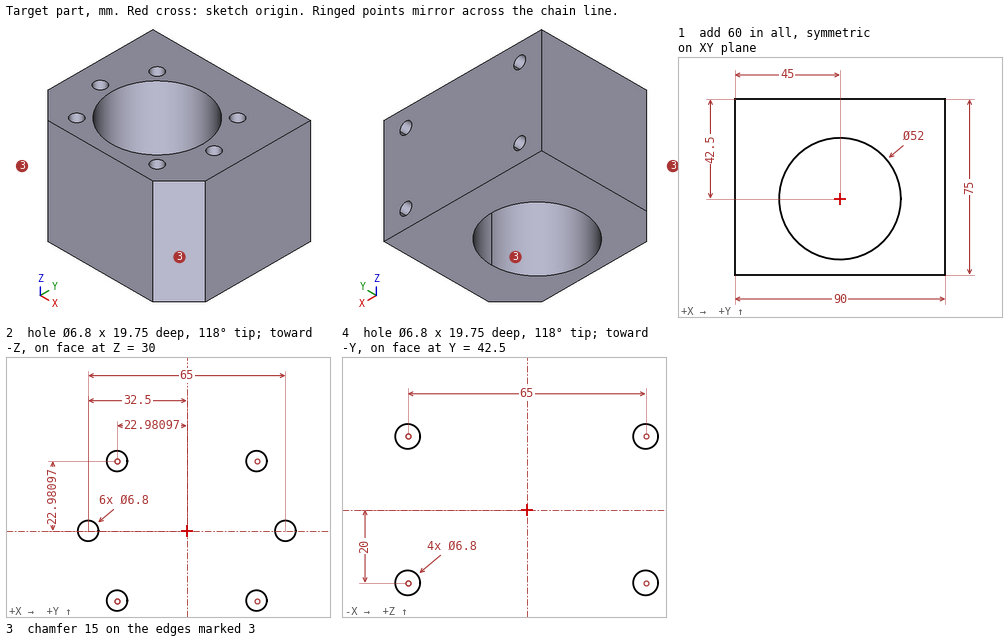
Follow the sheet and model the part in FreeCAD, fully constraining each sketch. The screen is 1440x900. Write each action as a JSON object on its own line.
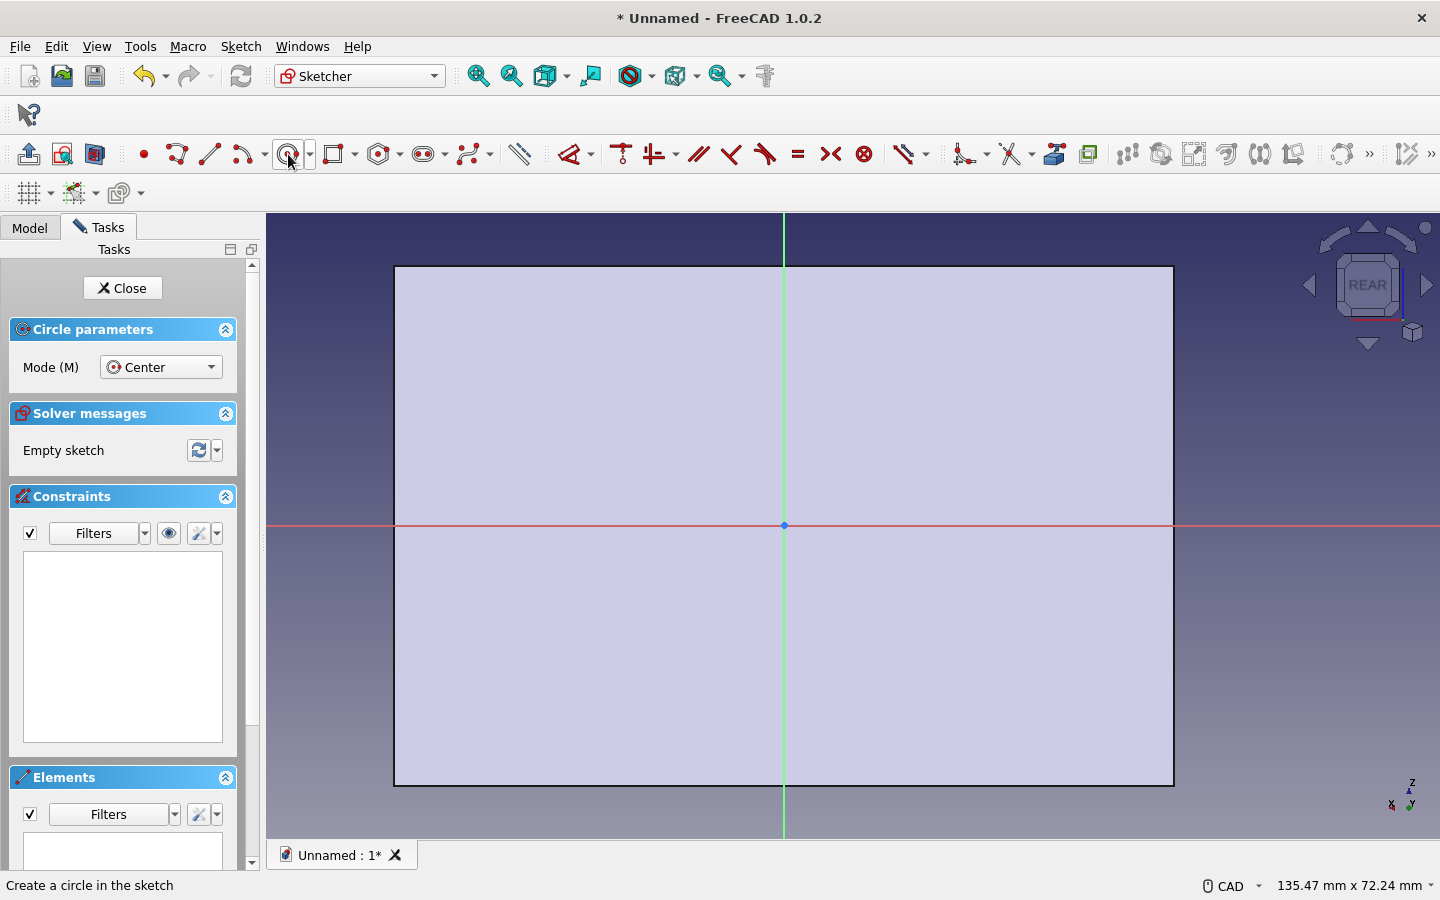
{"action": "left_click", "coordinate": [503, 699]}
{"action": "mouse_move", "coordinate": [523, 678]}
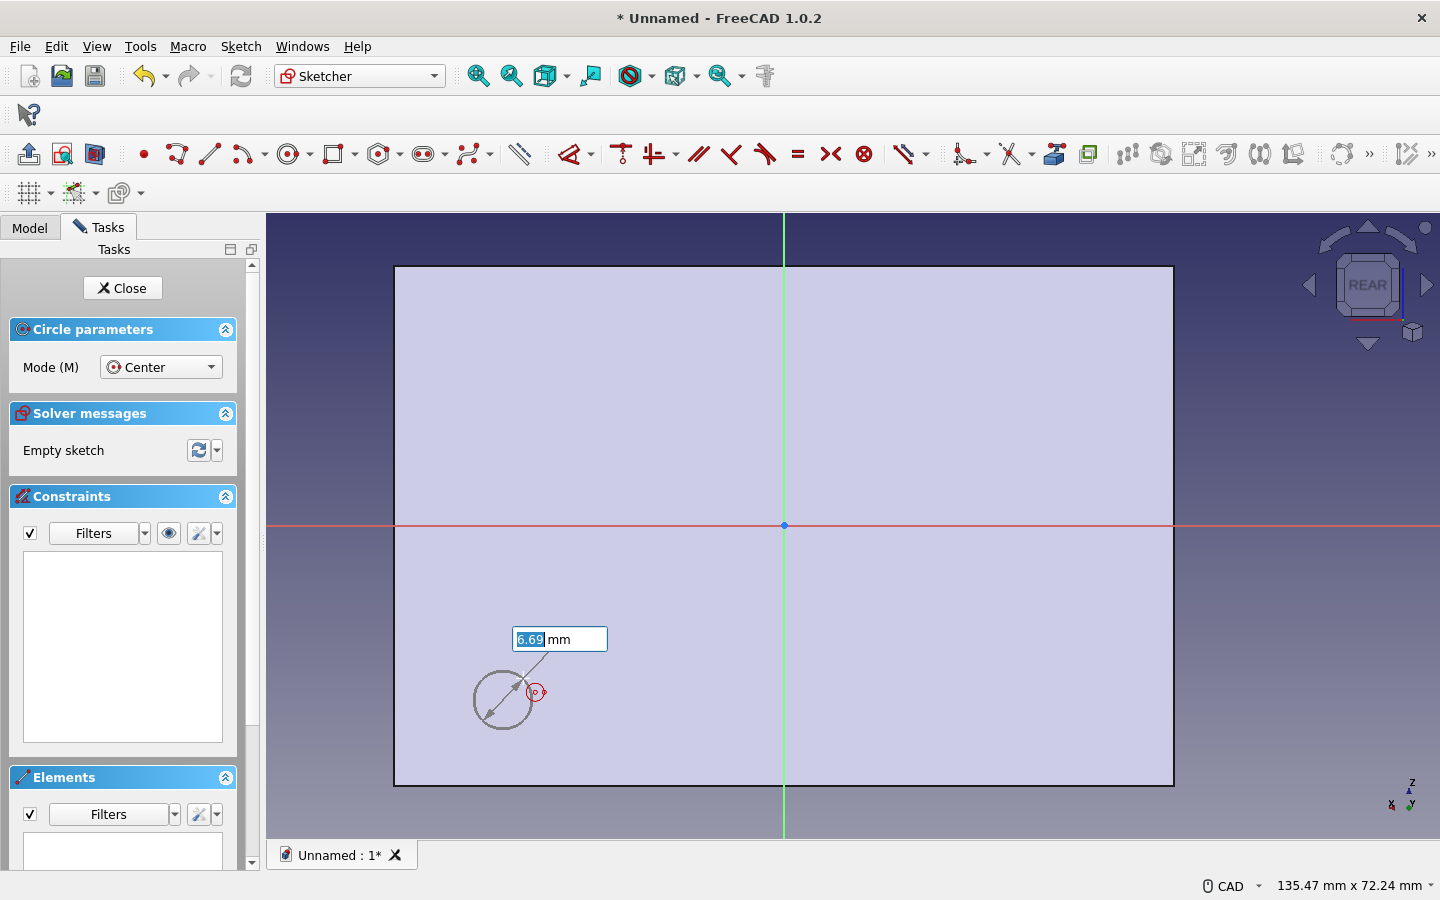
{"action": "type", "text": "6.8"}
{"action": "key", "text": "Return"}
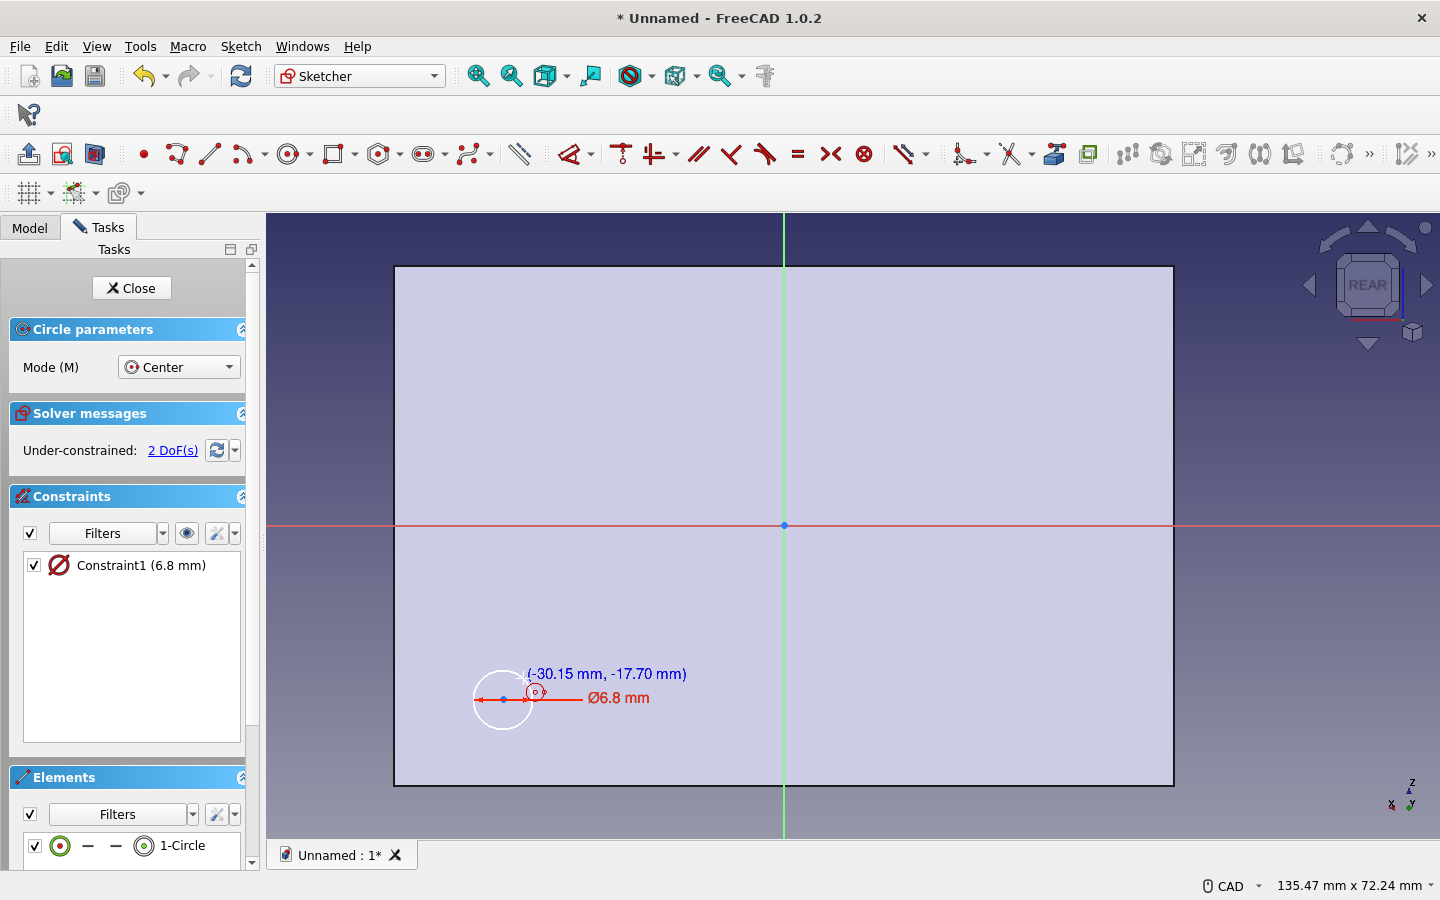
{"action": "left_click", "coordinate": [503, 352]}
{"action": "mouse_move", "coordinate": [523, 331]}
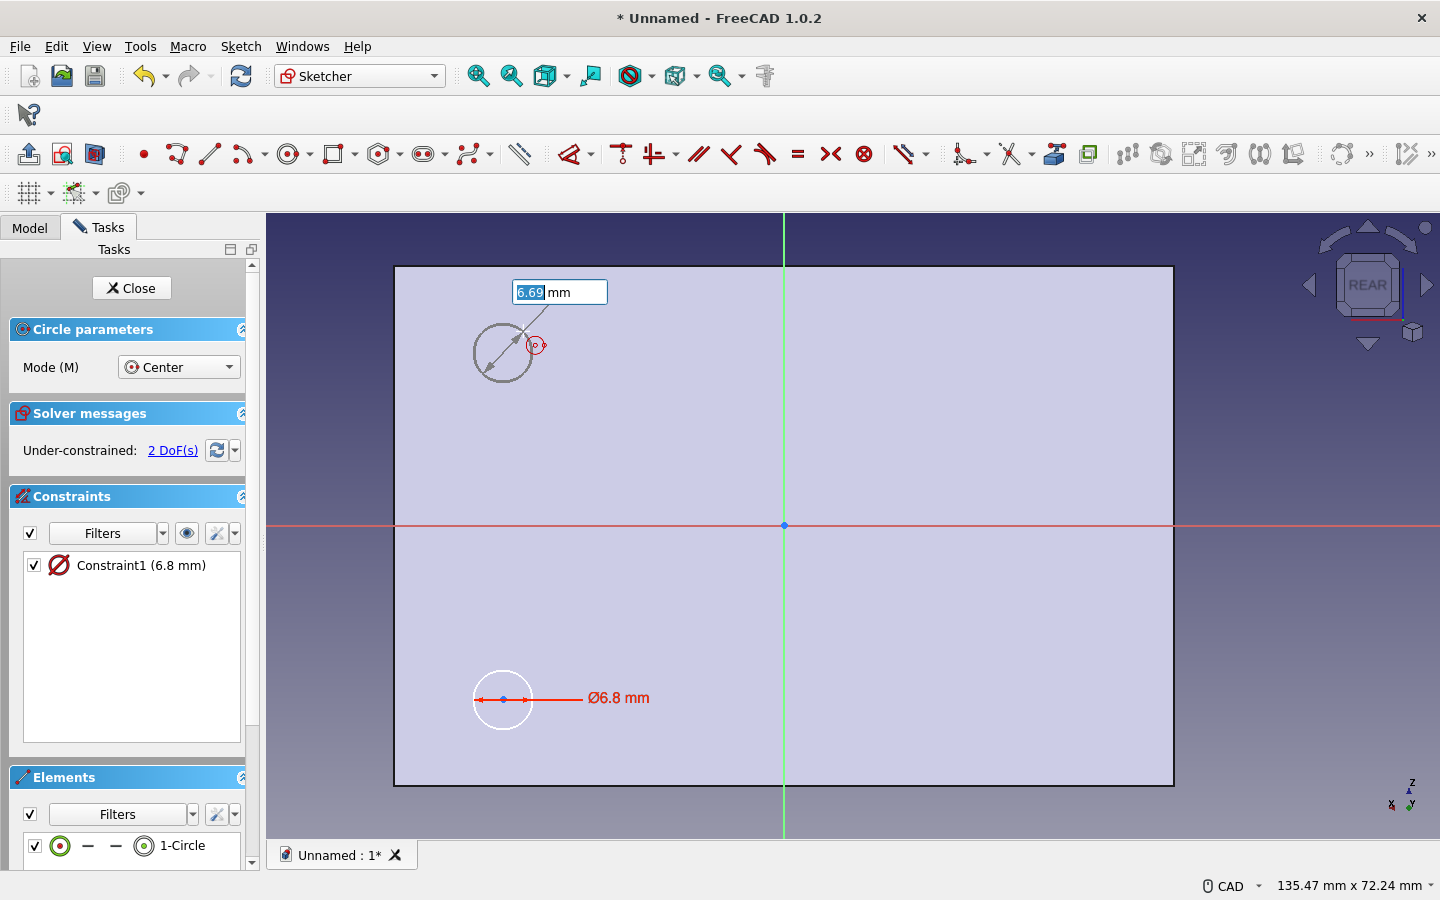
{"action": "type", "text": "6.8"}
{"action": "key", "text": "Return"}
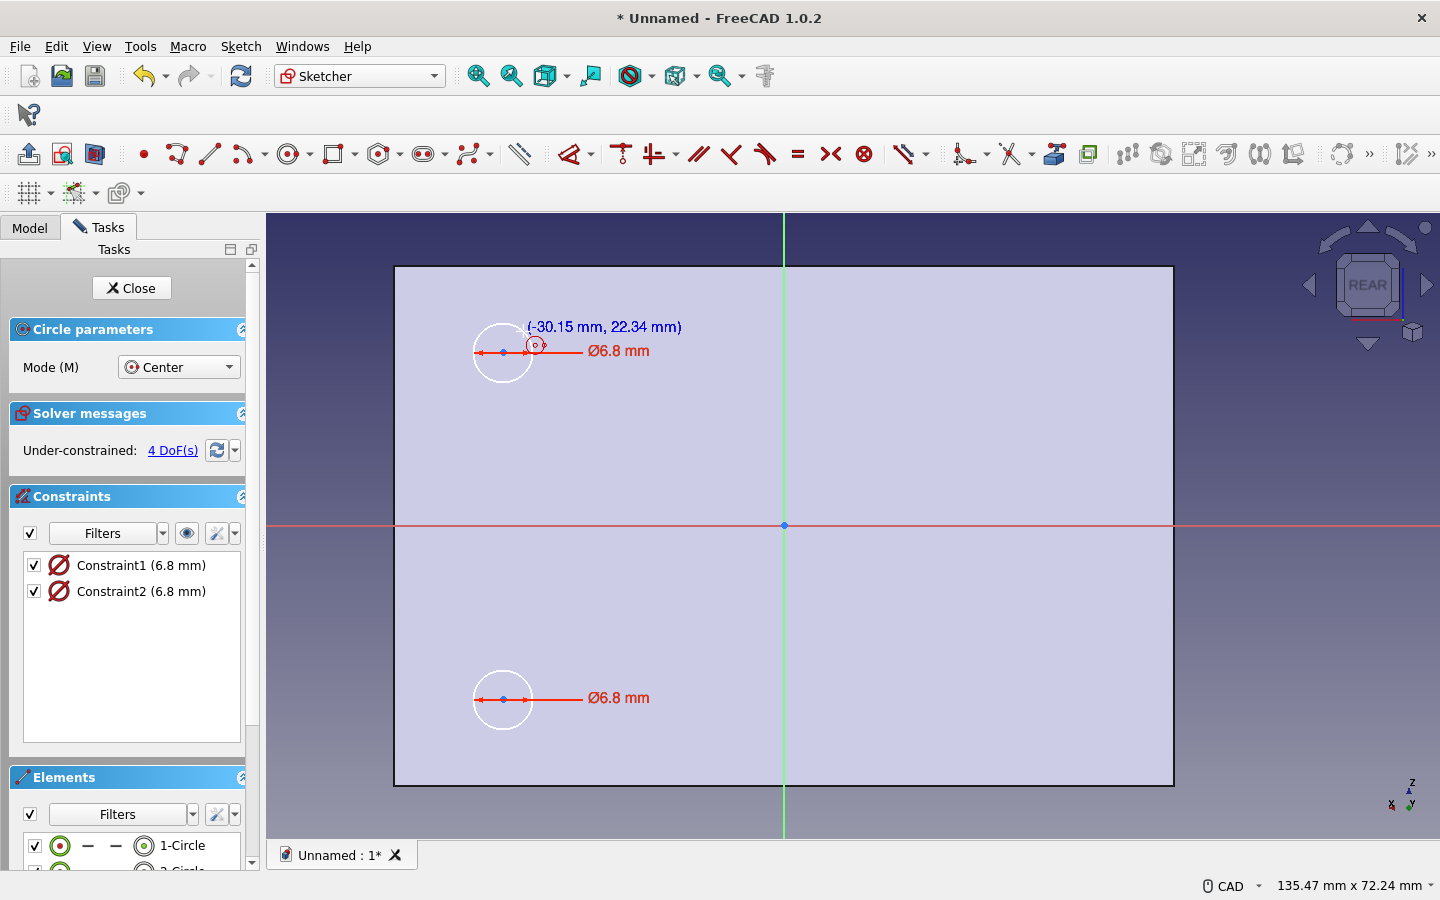
{"action": "left_click", "coordinate": [1066, 352]}
{"action": "mouse_move", "coordinate": [1087, 331]}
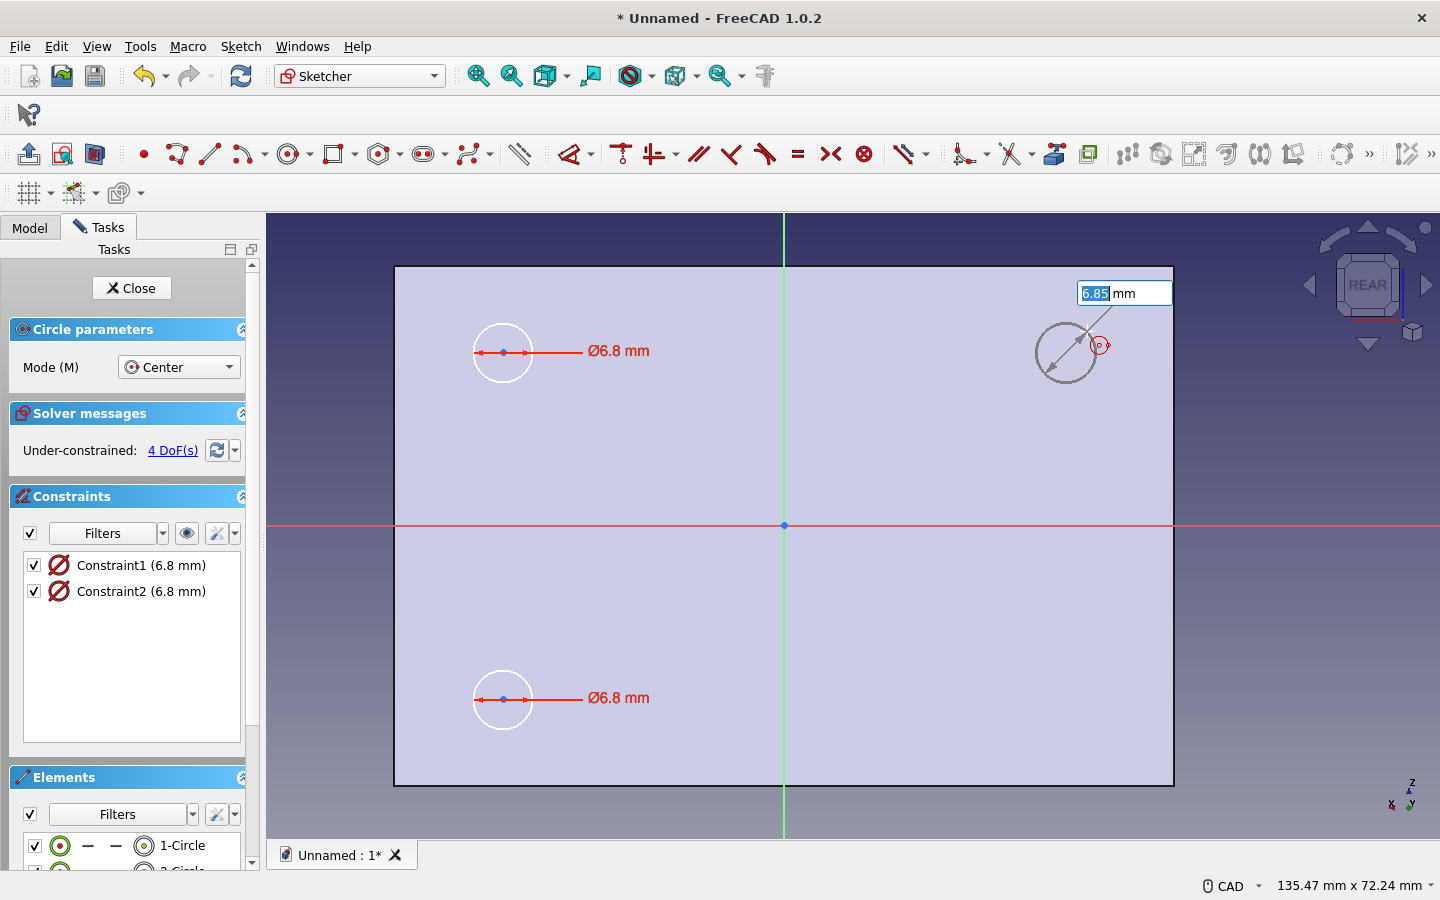
{"action": "type", "text": "6.8"}
{"action": "key", "text": "Return"}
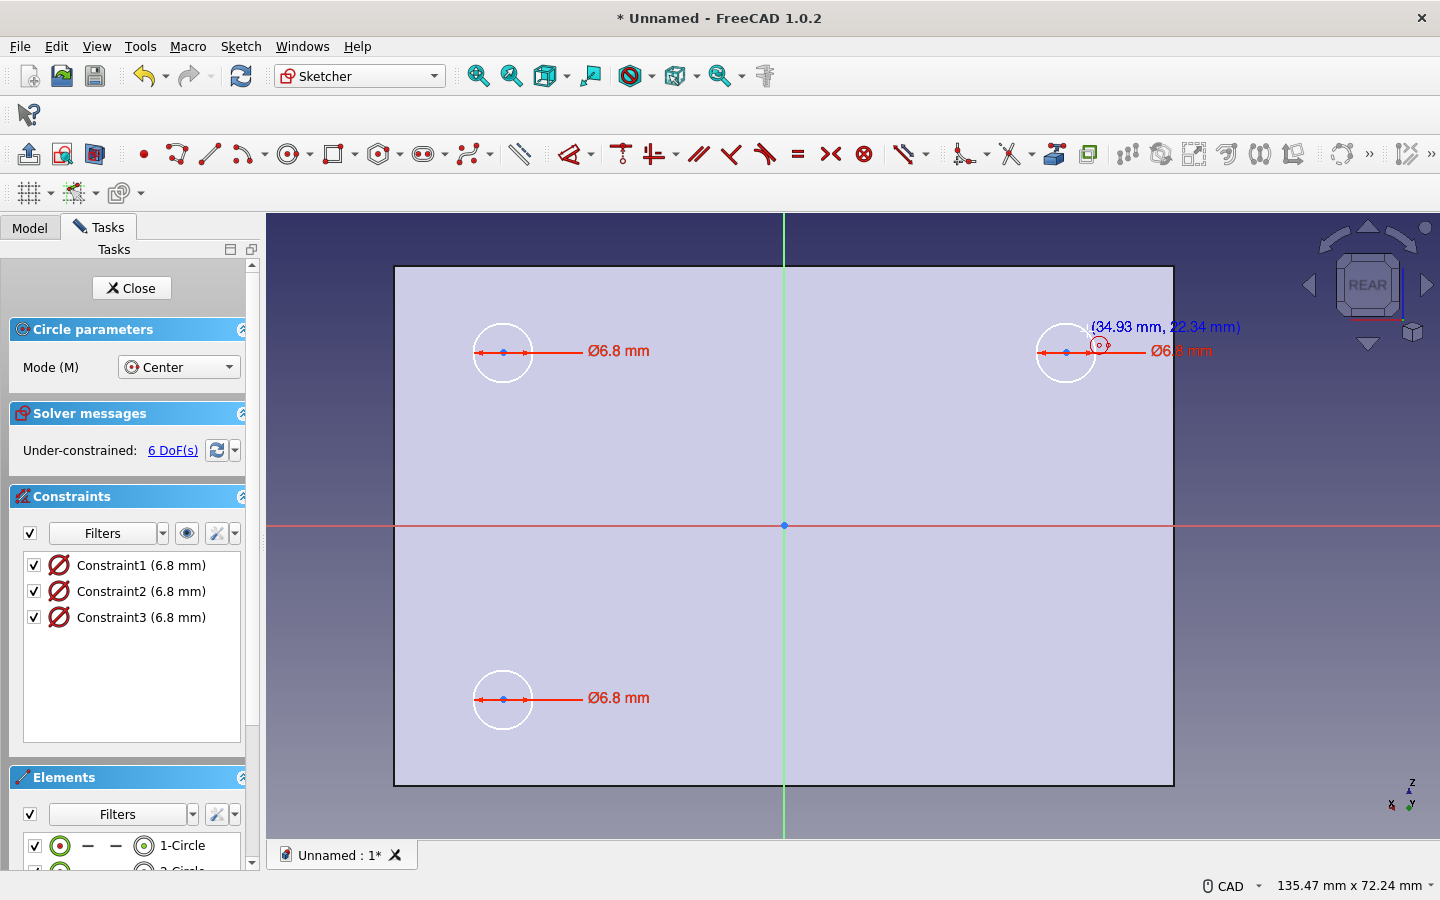
{"action": "left_click", "coordinate": [1066, 699]}
{"action": "mouse_move", "coordinate": [1087, 678]}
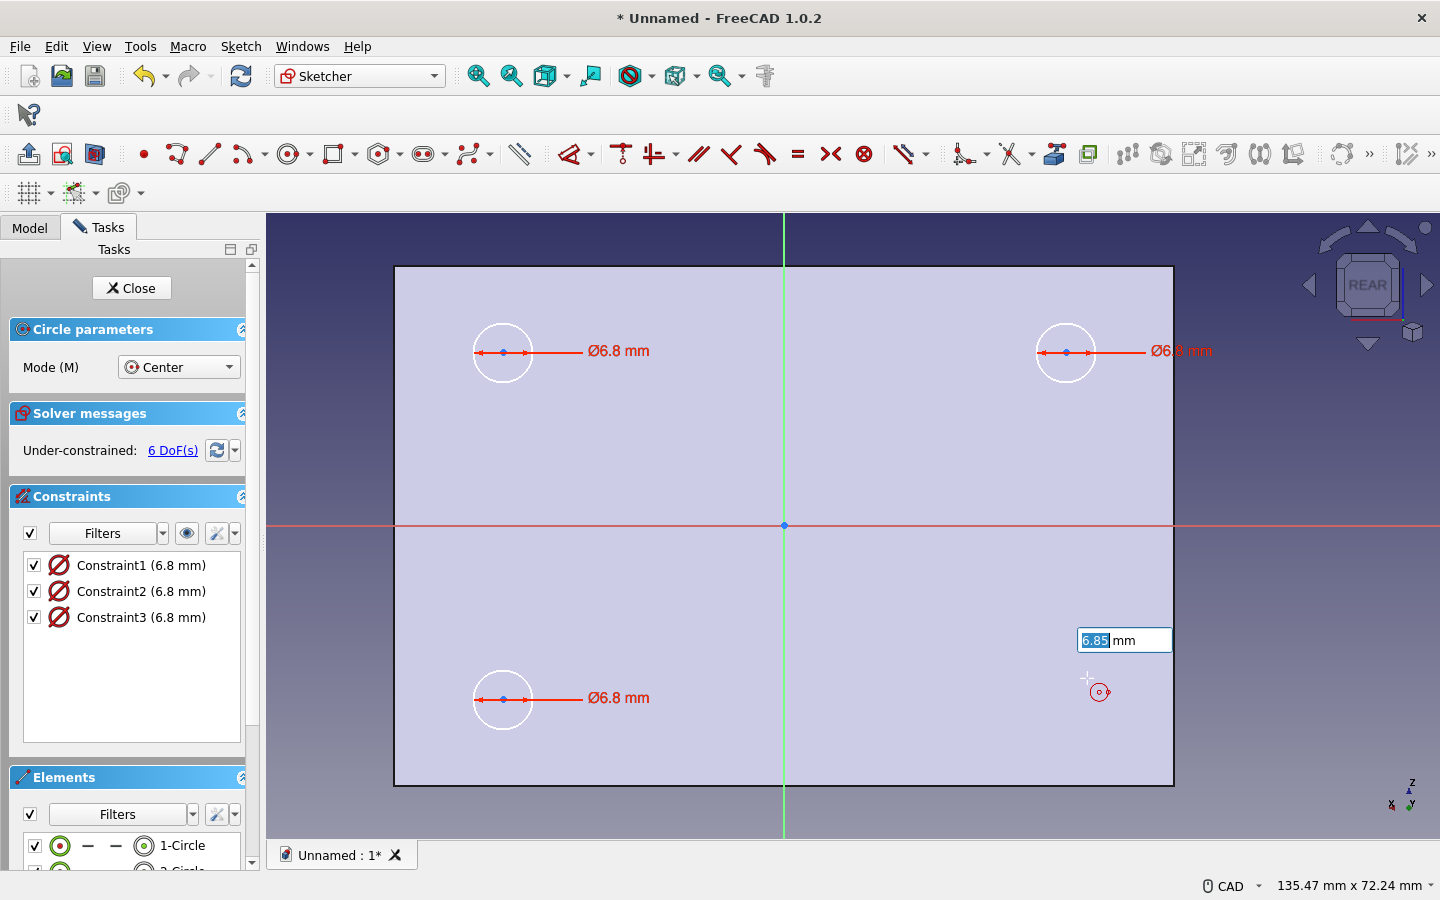
{"action": "type", "text": "6.8"}
{"action": "key", "text": "Return"}
{"action": "key", "text": "Escape"}